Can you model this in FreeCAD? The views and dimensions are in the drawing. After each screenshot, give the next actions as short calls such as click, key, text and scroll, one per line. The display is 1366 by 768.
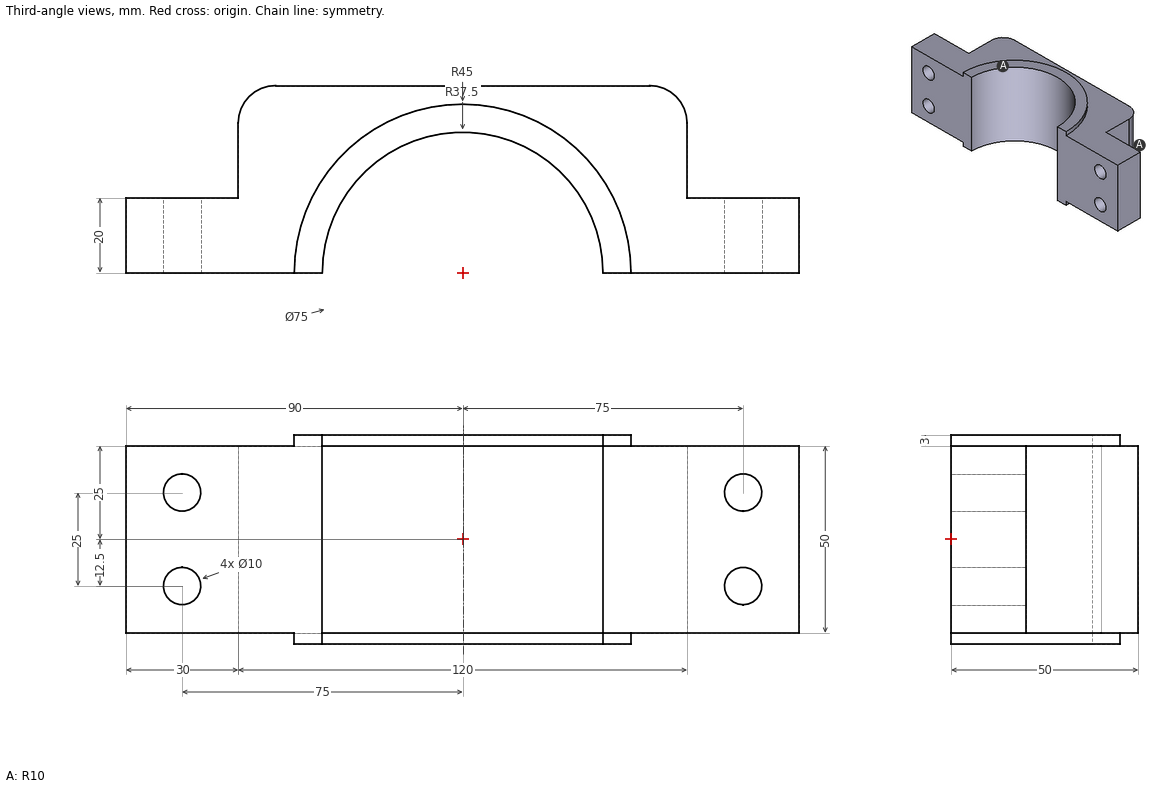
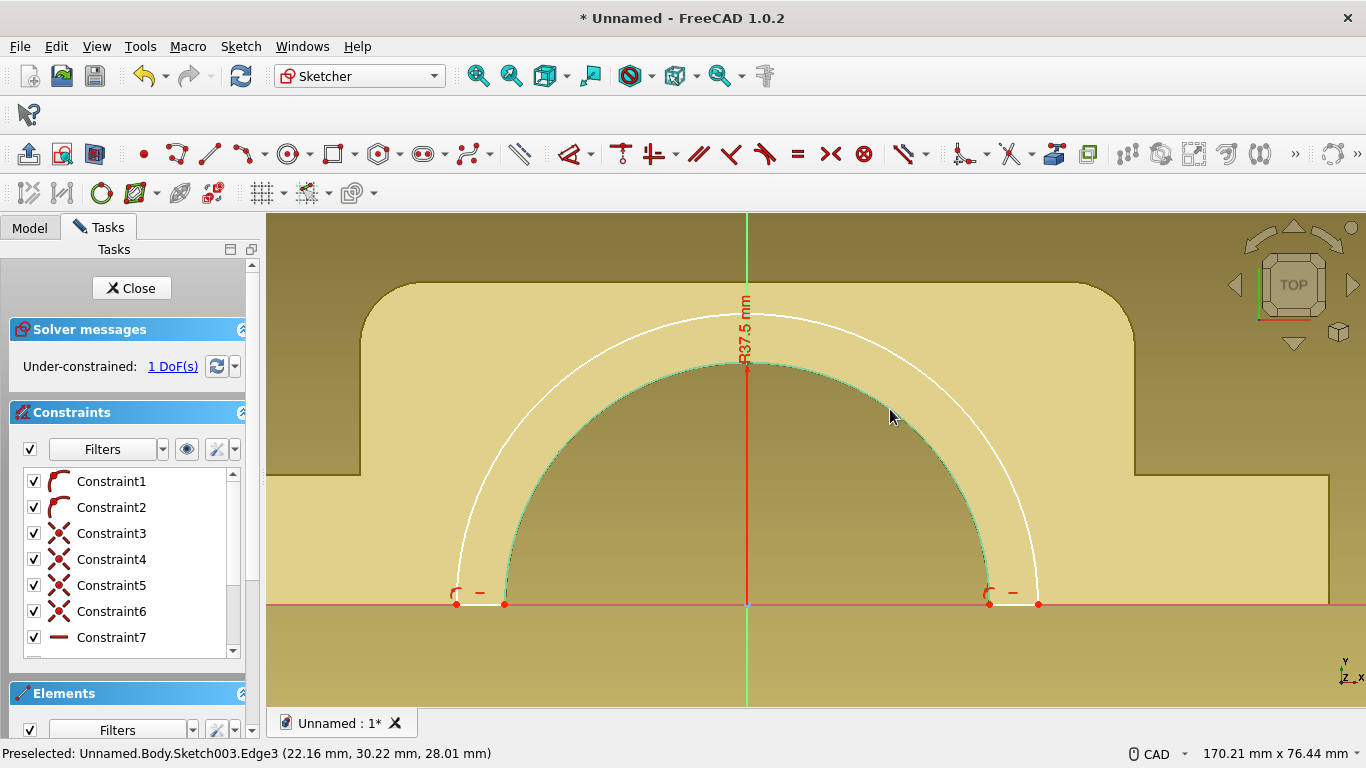
click(918, 369)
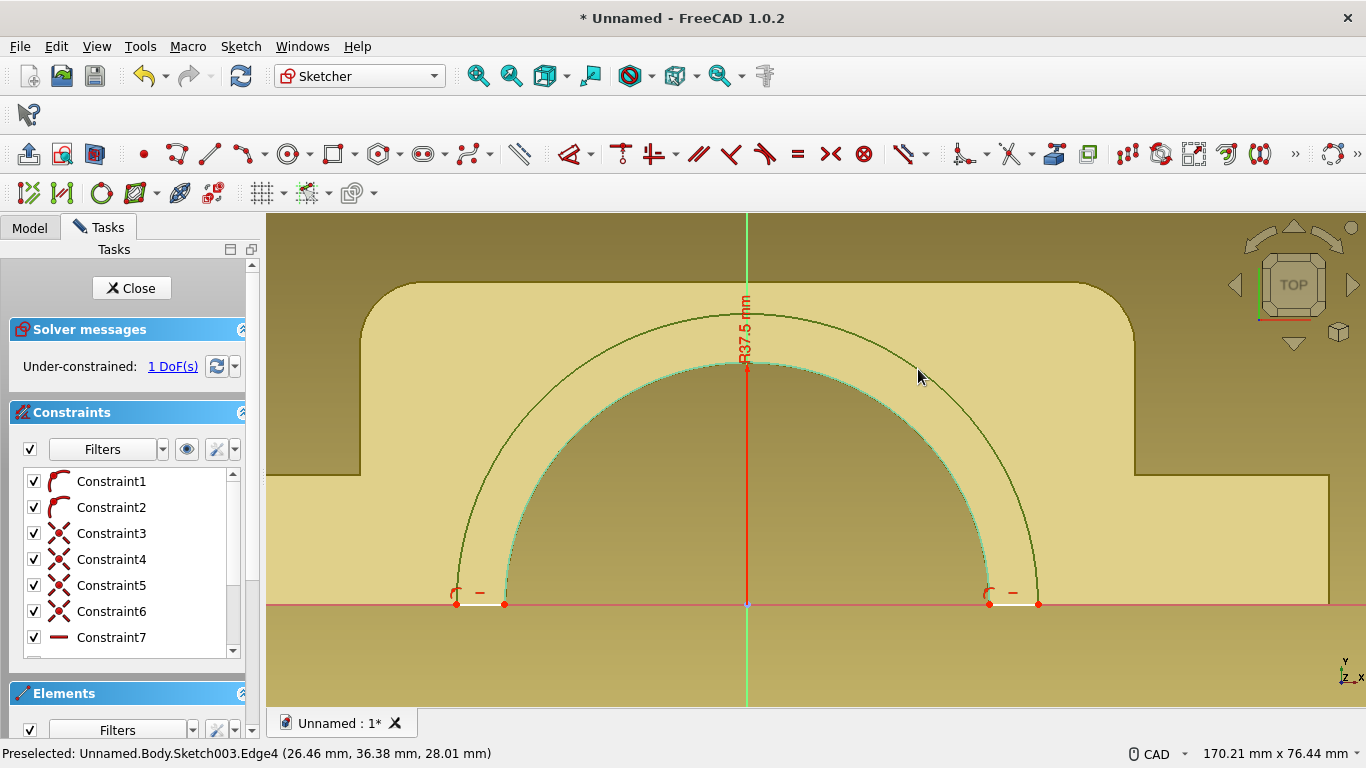
key(k)
key(r)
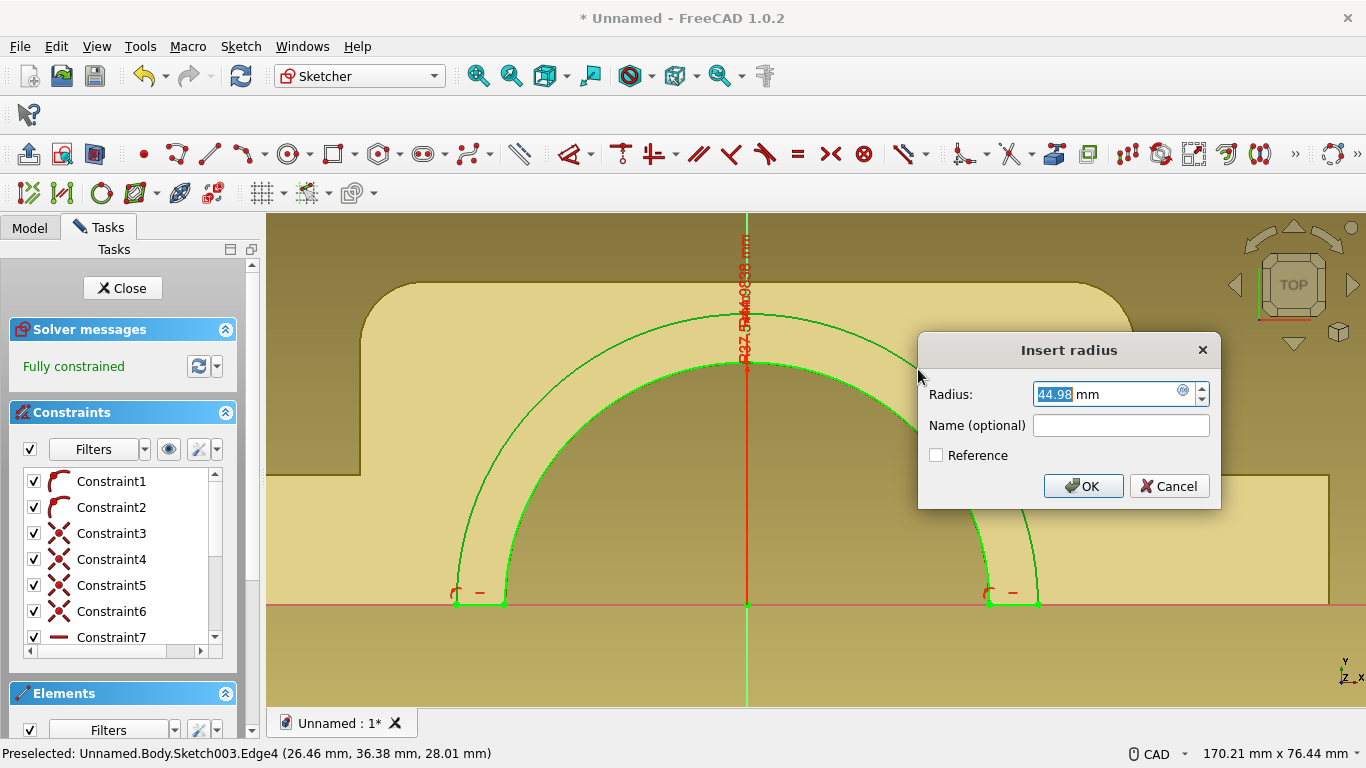
text(45)
key(Return)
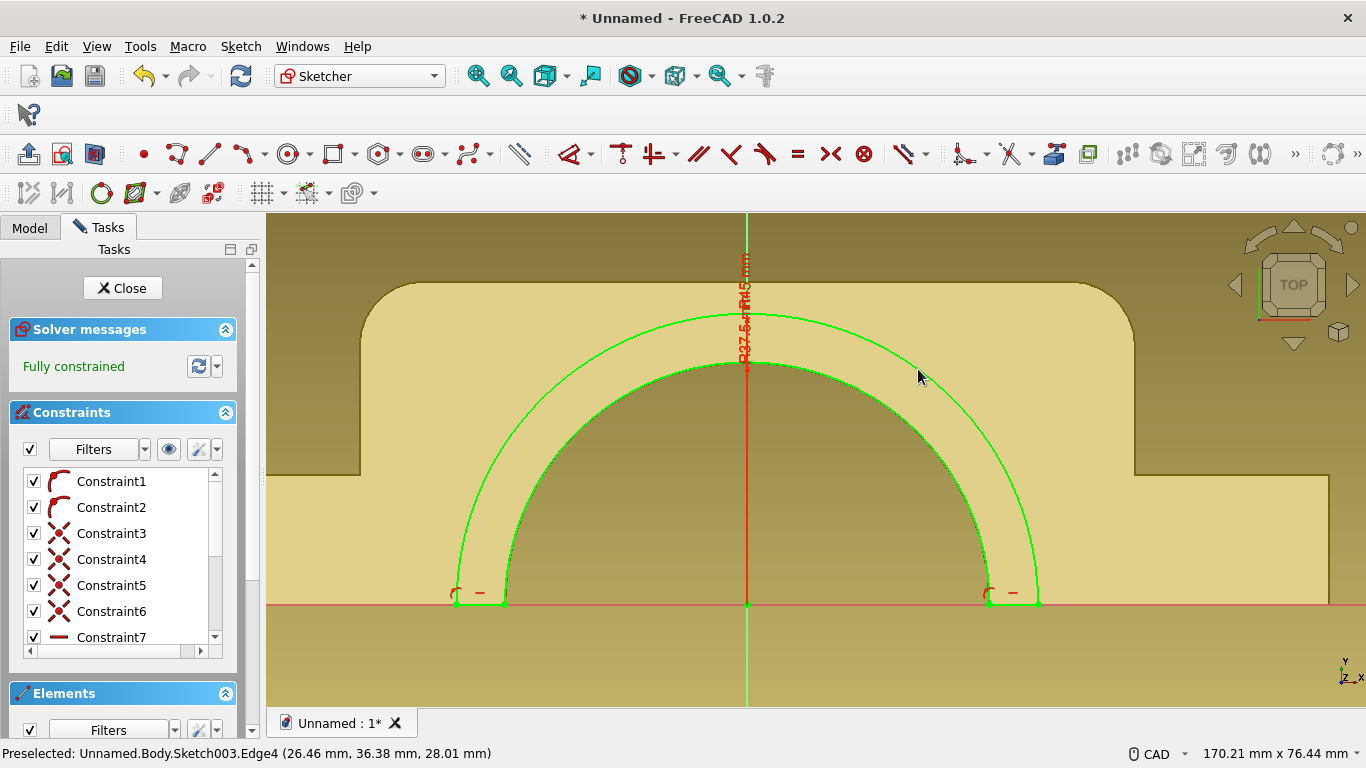
click(123, 288)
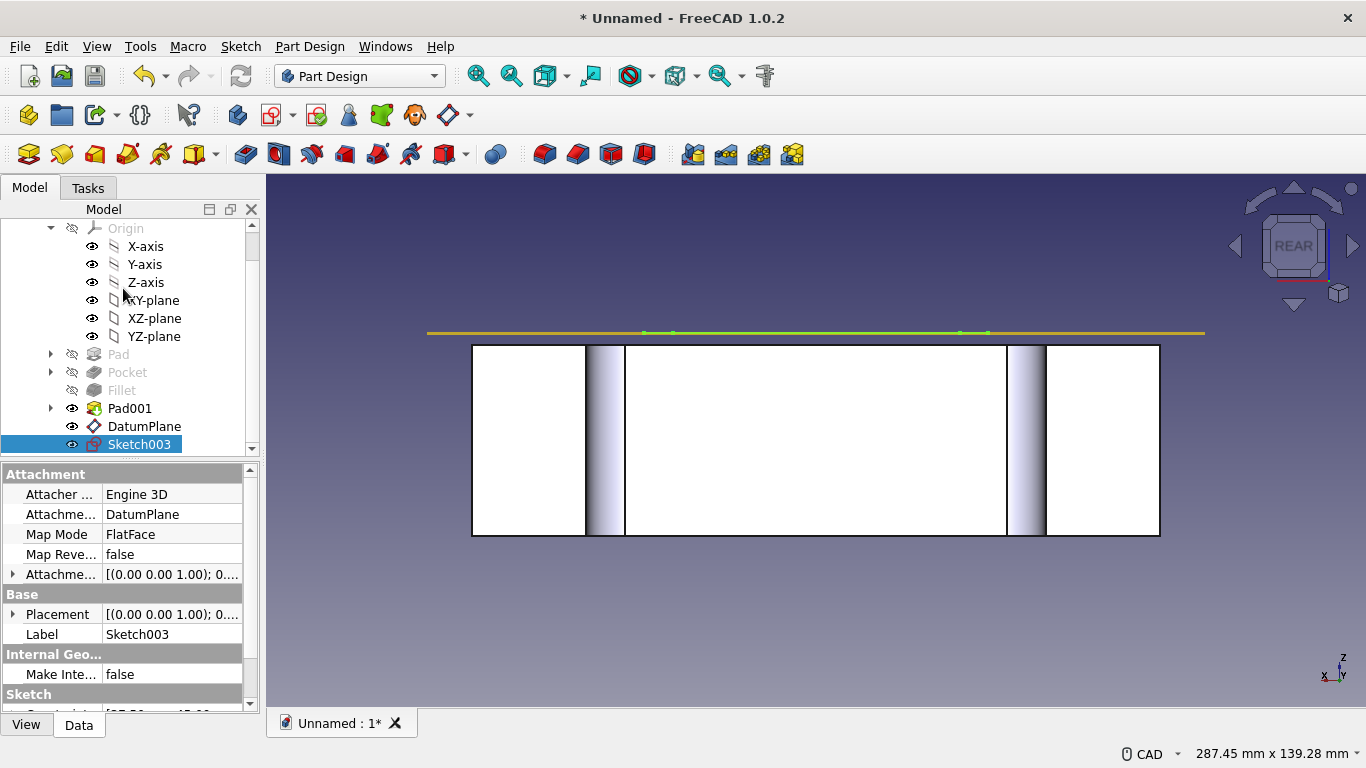
click(29, 154)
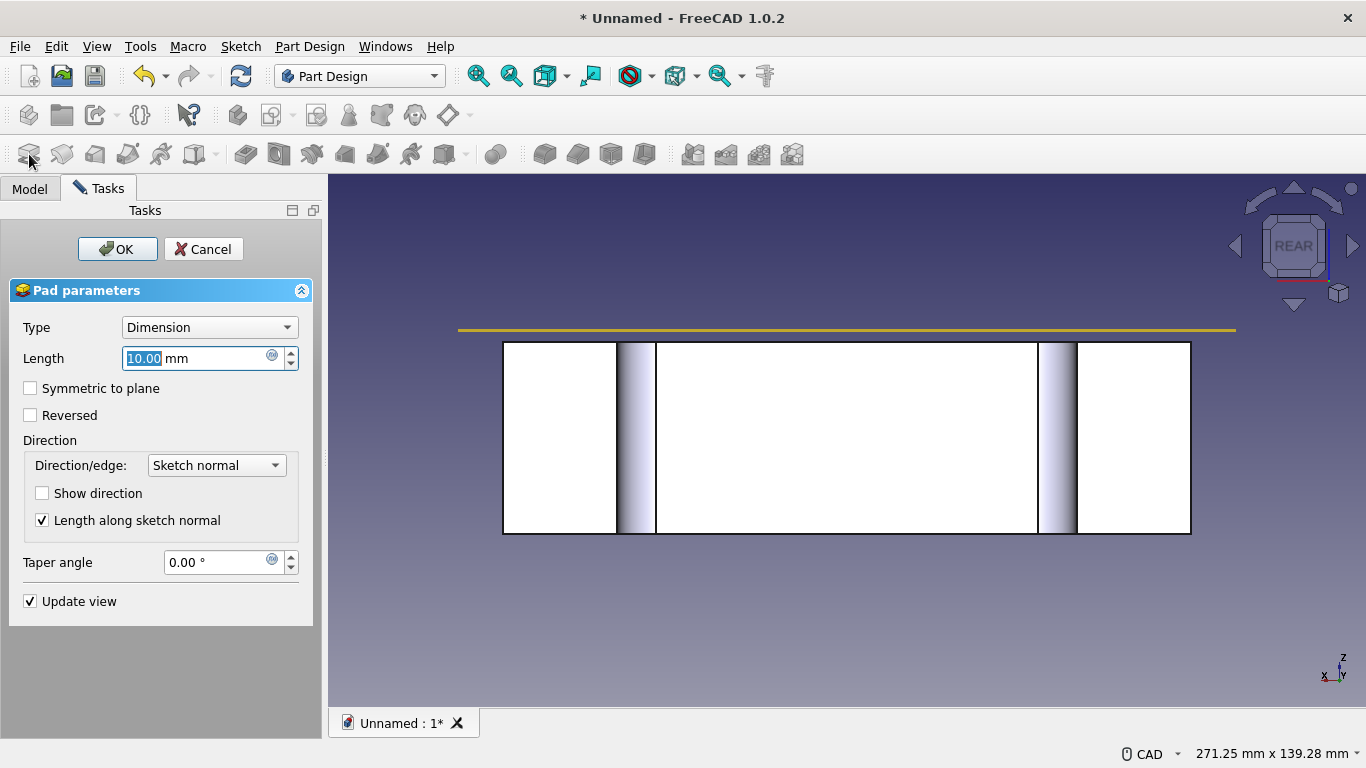
text(3)
key(Tab)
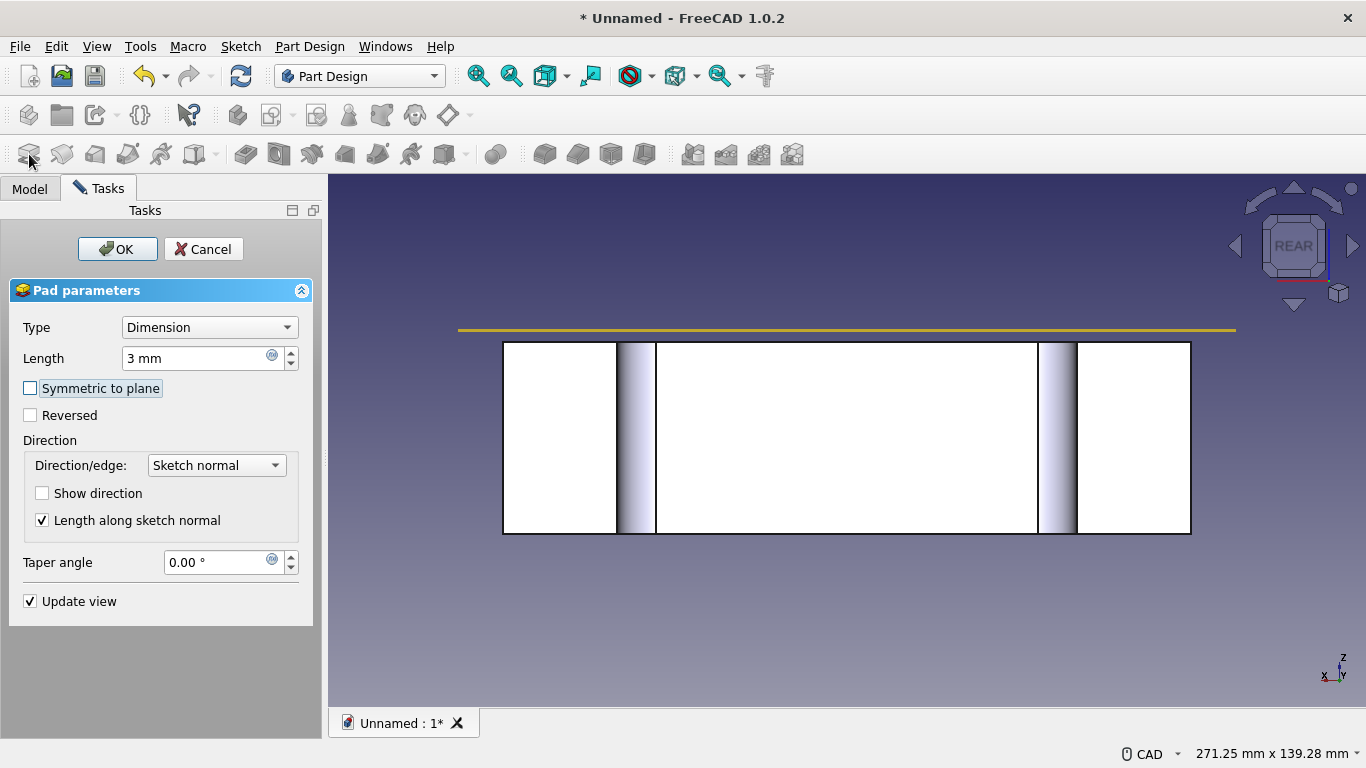
click(31, 415)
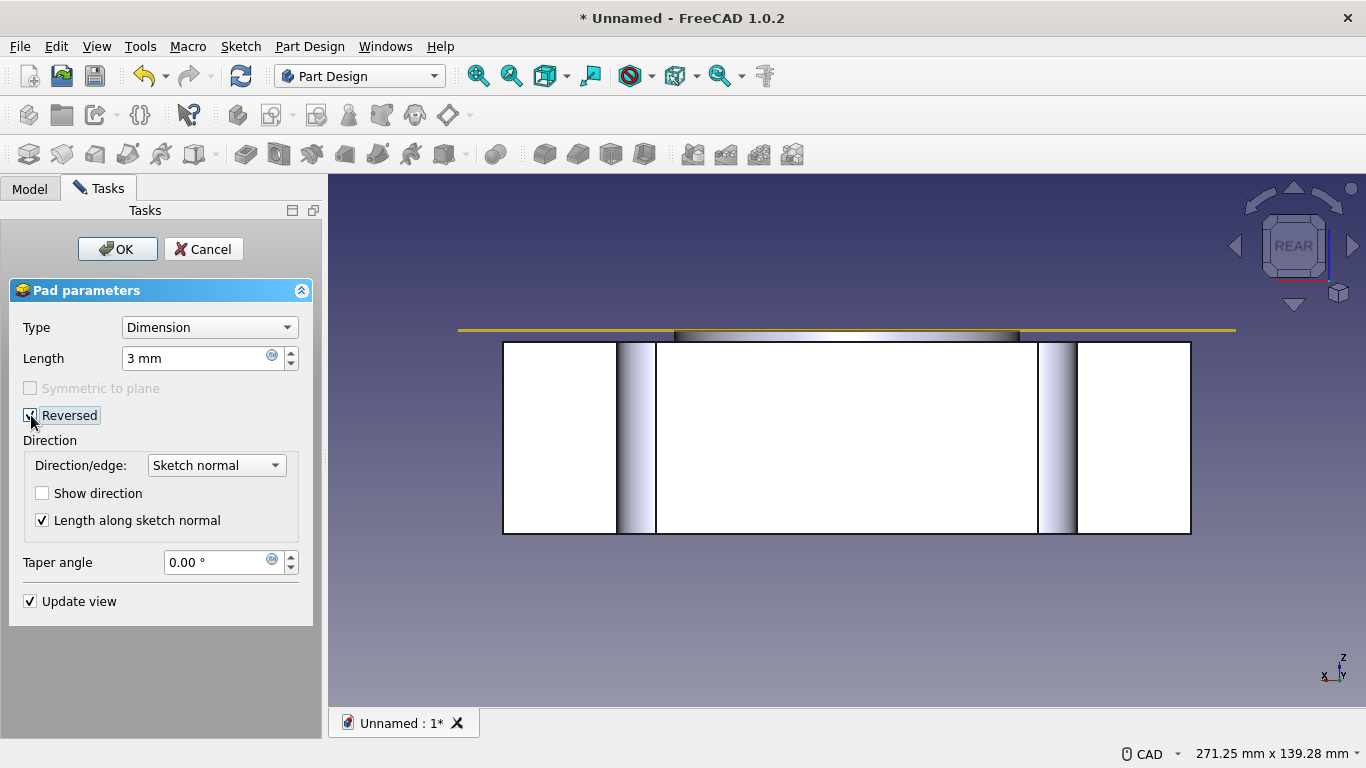
click(118, 249)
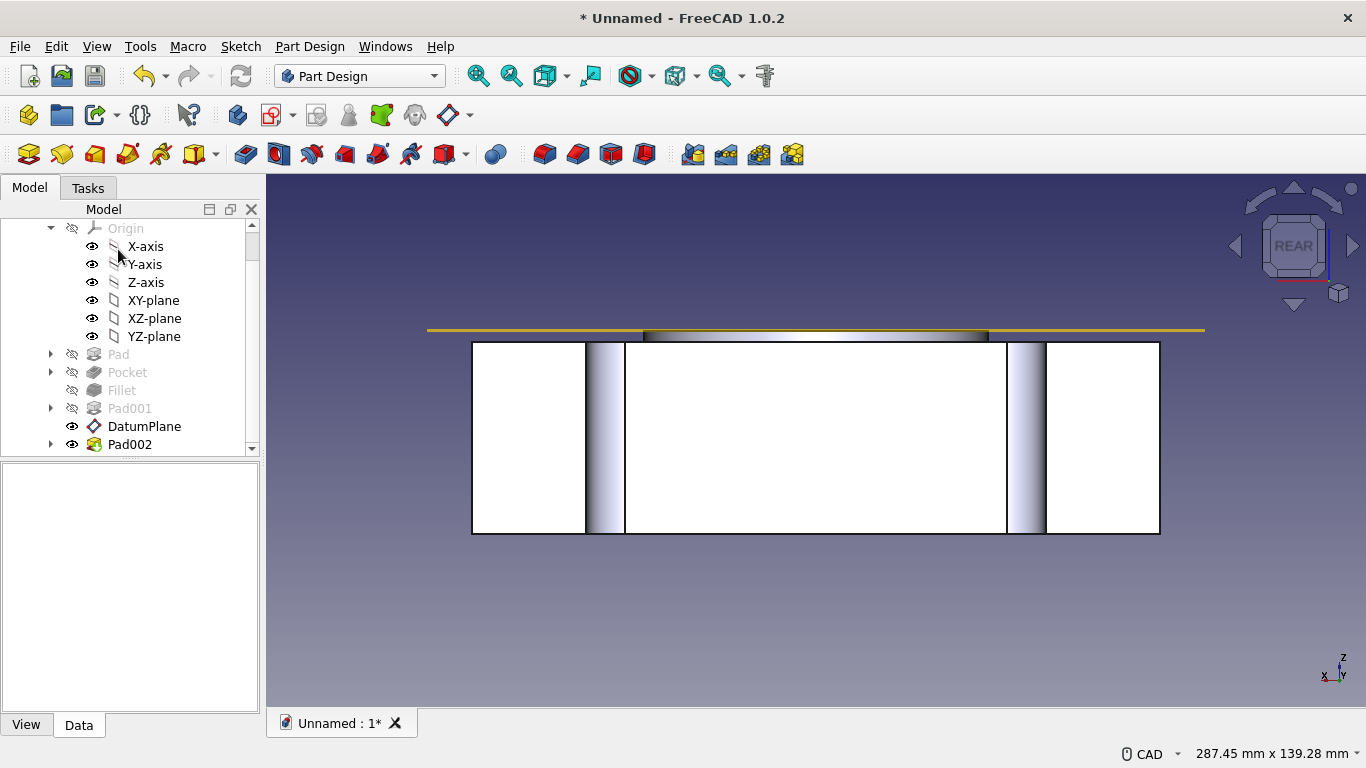
click(117, 426)
key(space)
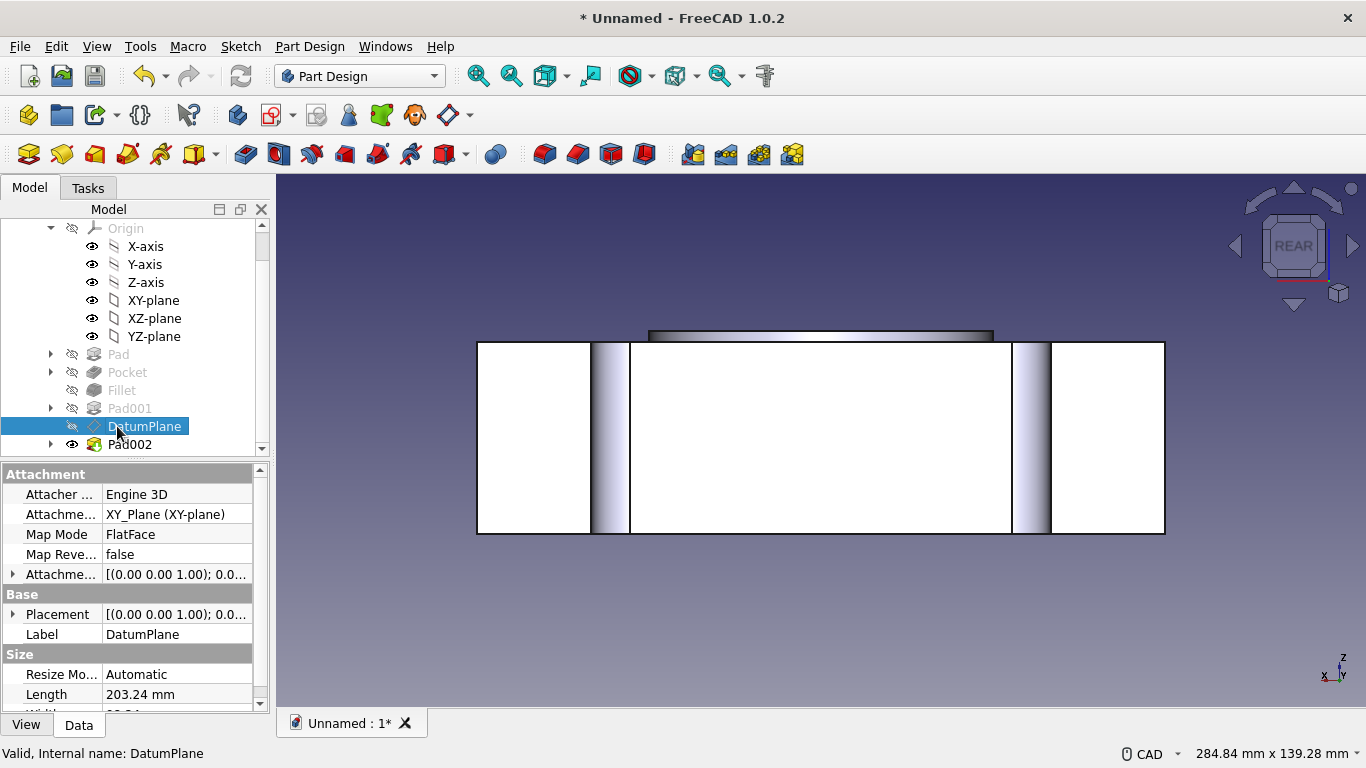
click(117, 444)